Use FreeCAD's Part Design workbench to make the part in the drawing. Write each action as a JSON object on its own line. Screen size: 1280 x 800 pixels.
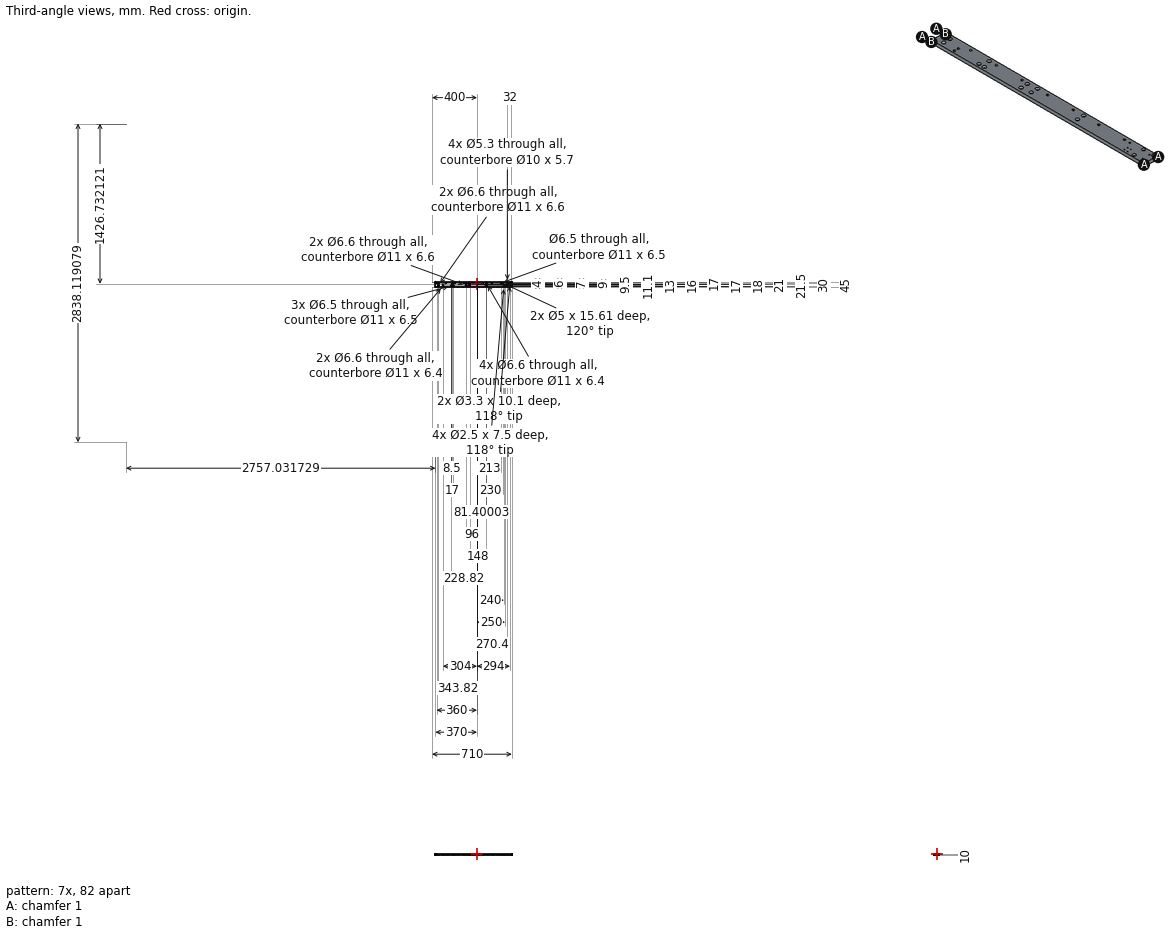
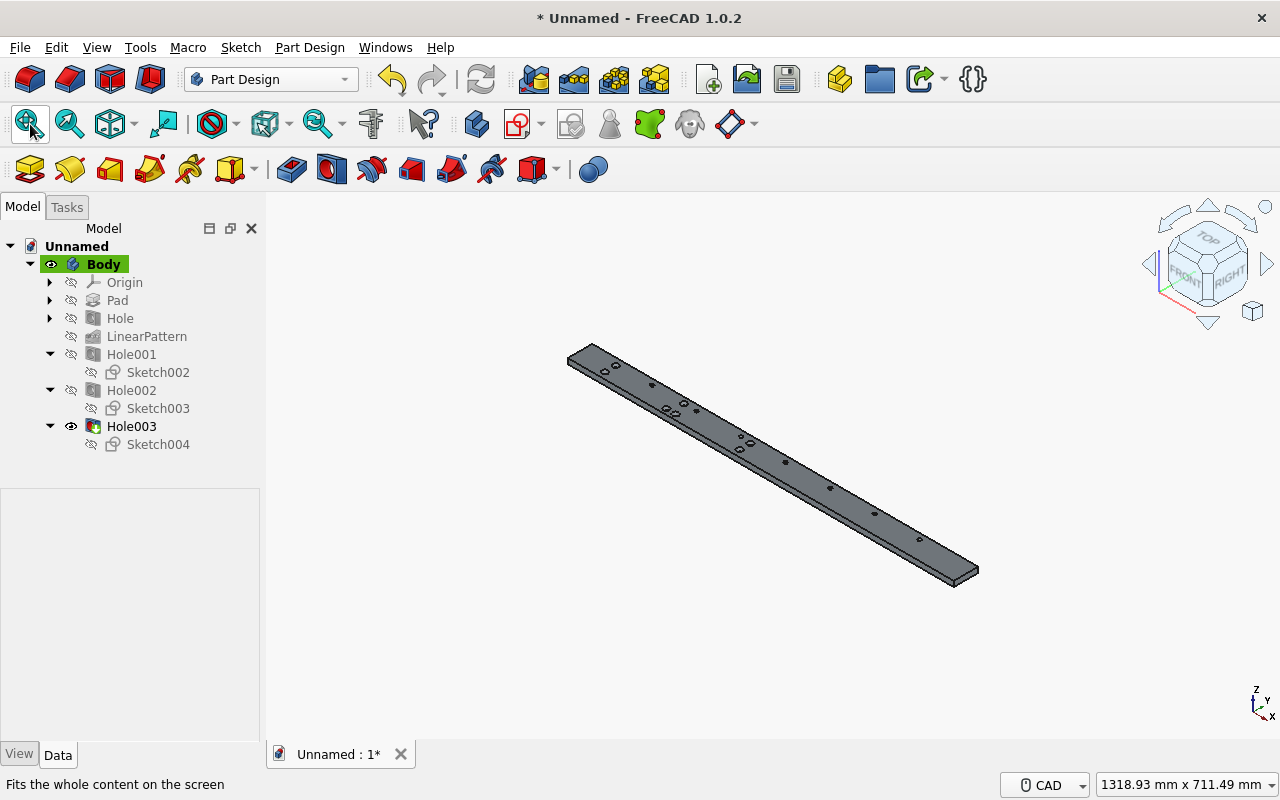
{"action": "key", "text": "5"}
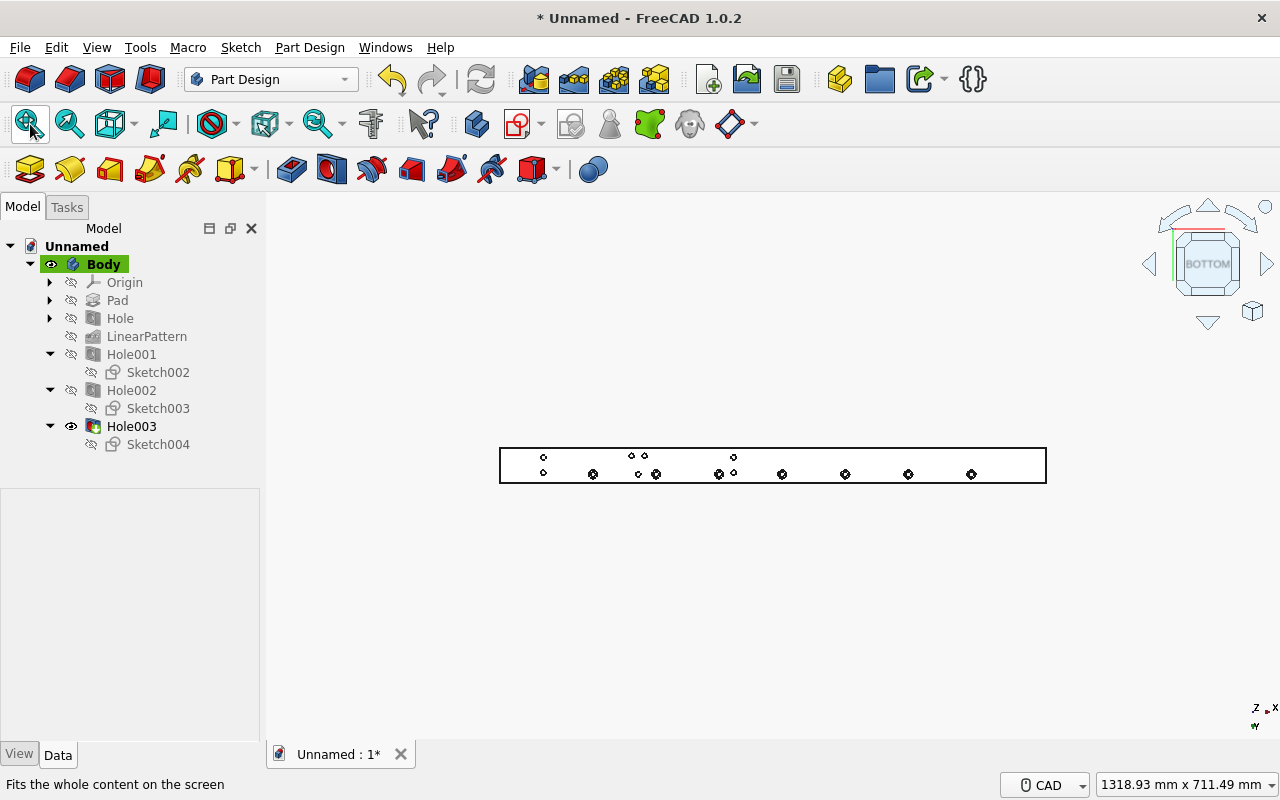
{"action": "left_click", "coordinate": [1007, 464]}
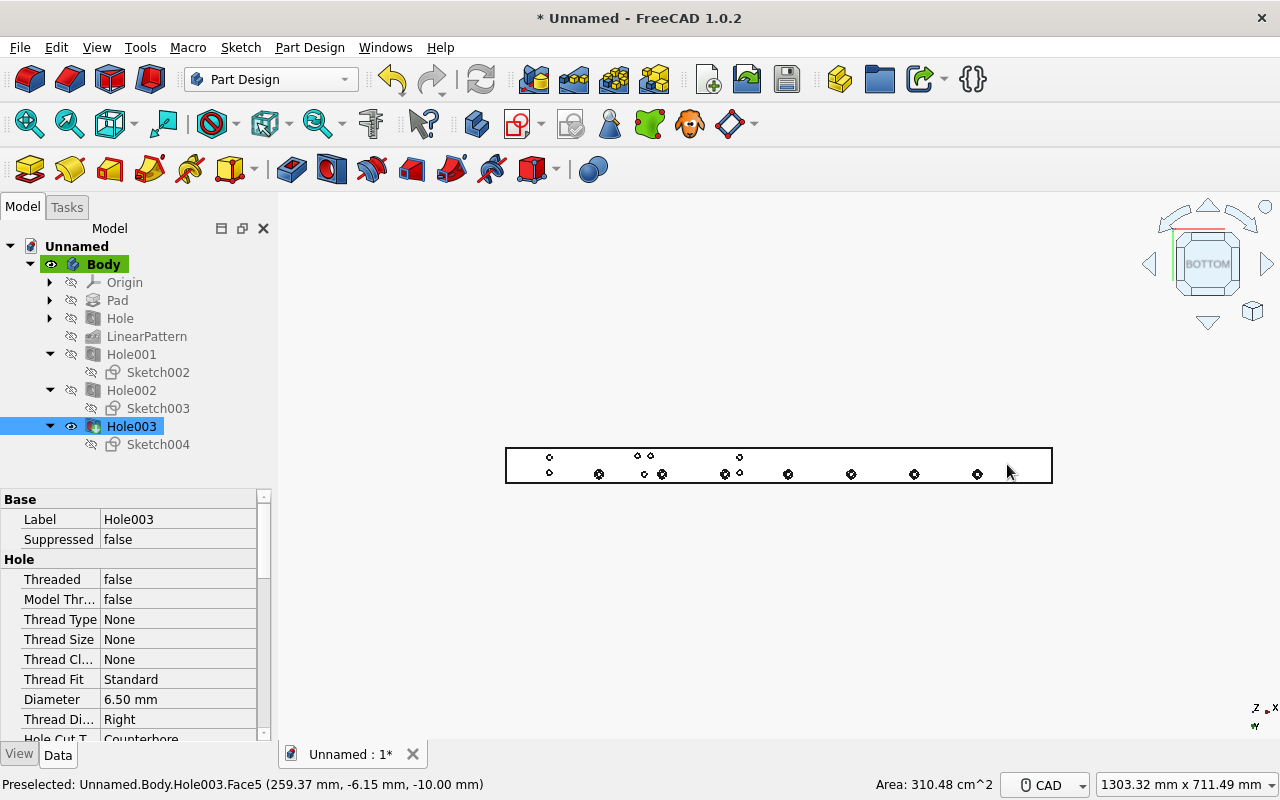
{"action": "left_click", "coordinate": [518, 124]}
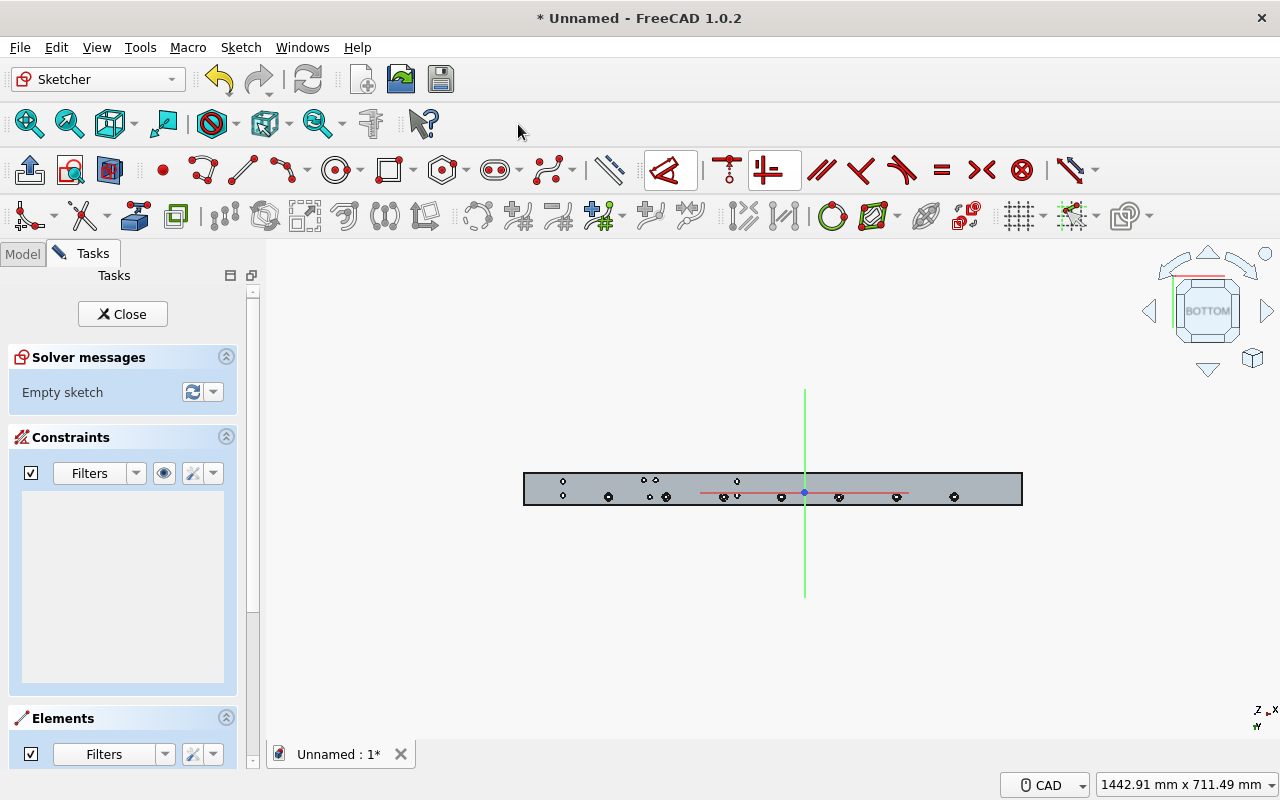
{"action": "scroll", "coordinate": [585, 482], "scroll_direction": "up", "scroll_amount": 15}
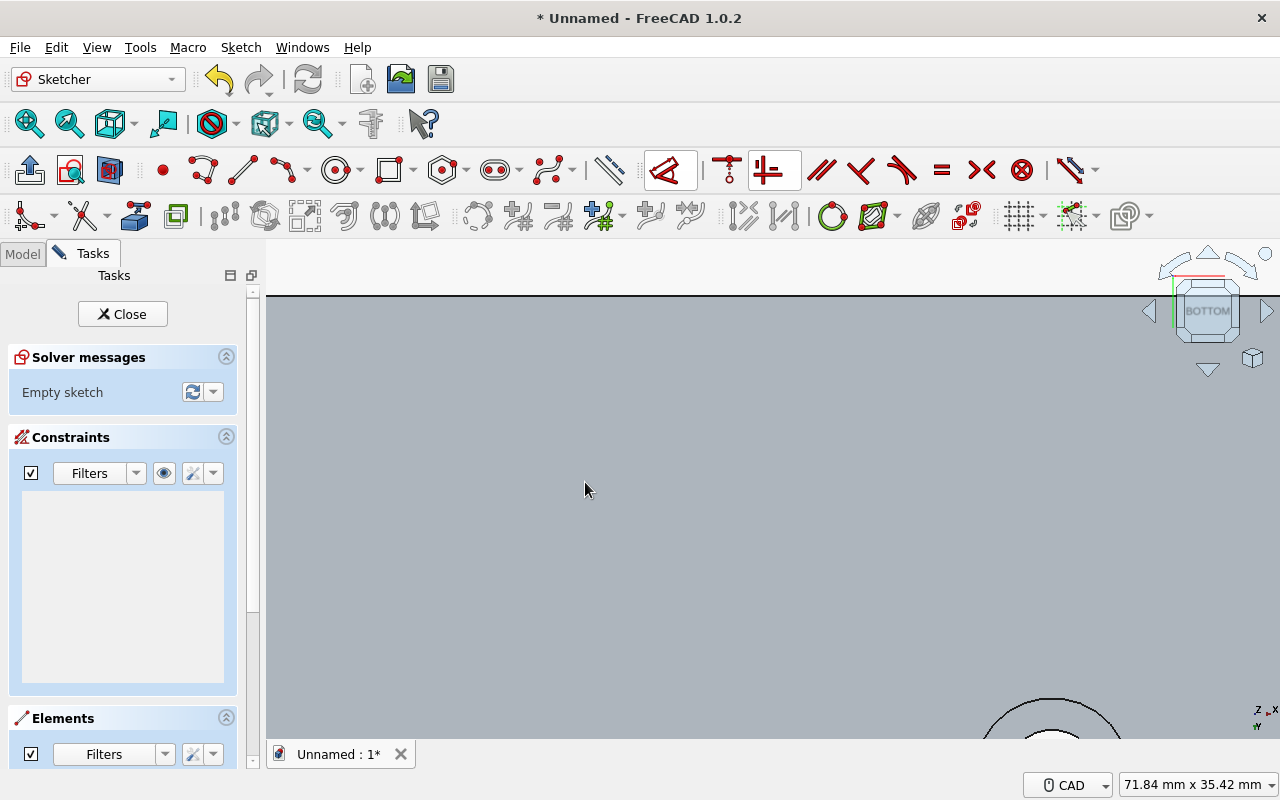
{"action": "left_click", "coordinate": [336, 170]}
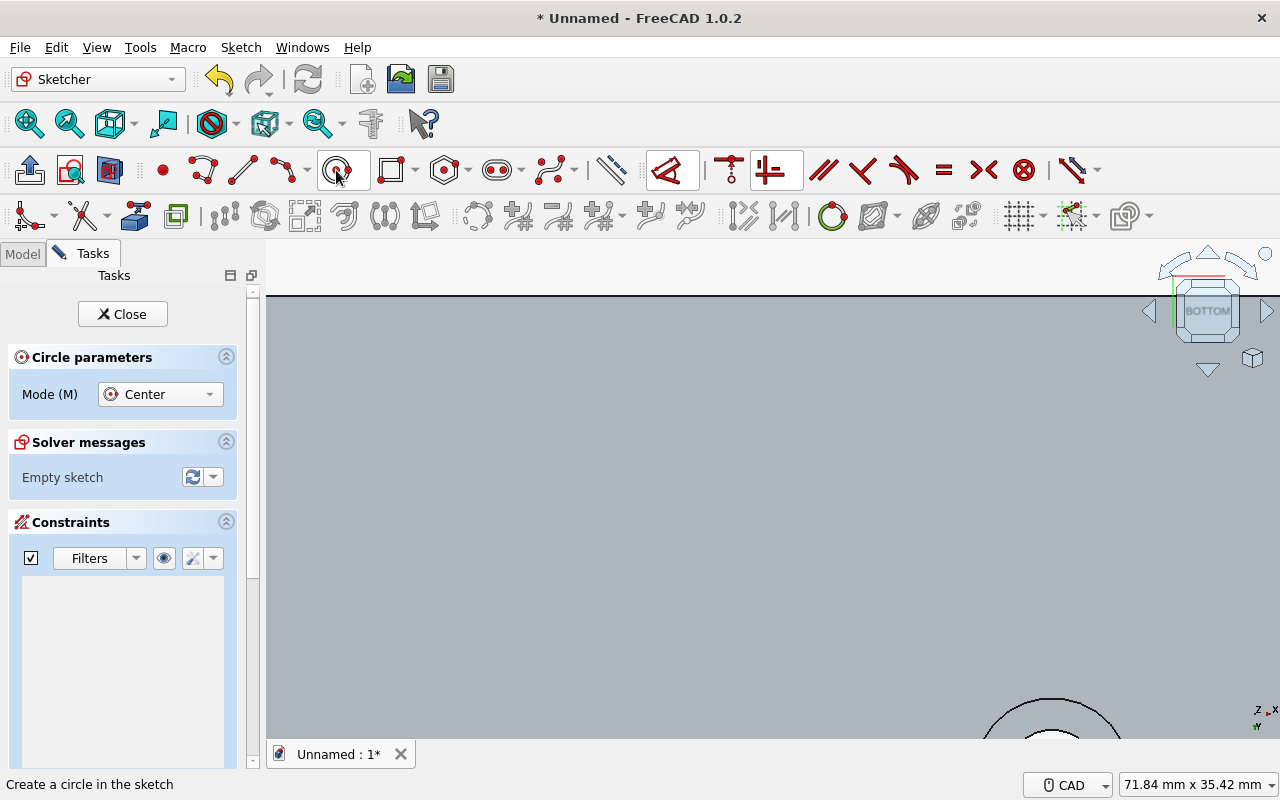
{"action": "left_click", "coordinate": [699, 395]}
{"action": "left_click", "coordinate": [732, 362]}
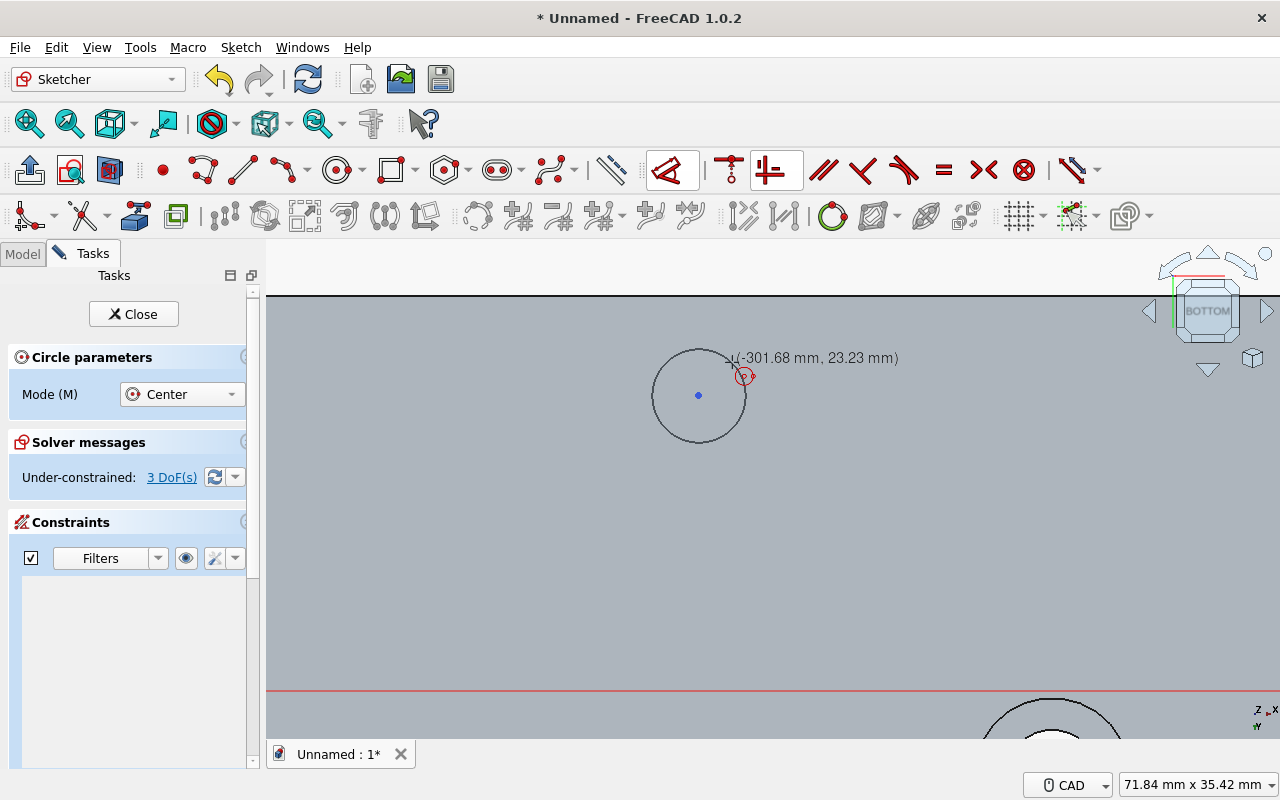
{"action": "left_click", "coordinate": [699, 564]}
{"action": "left_click", "coordinate": [732, 531]}
{"action": "key", "text": "Escape"}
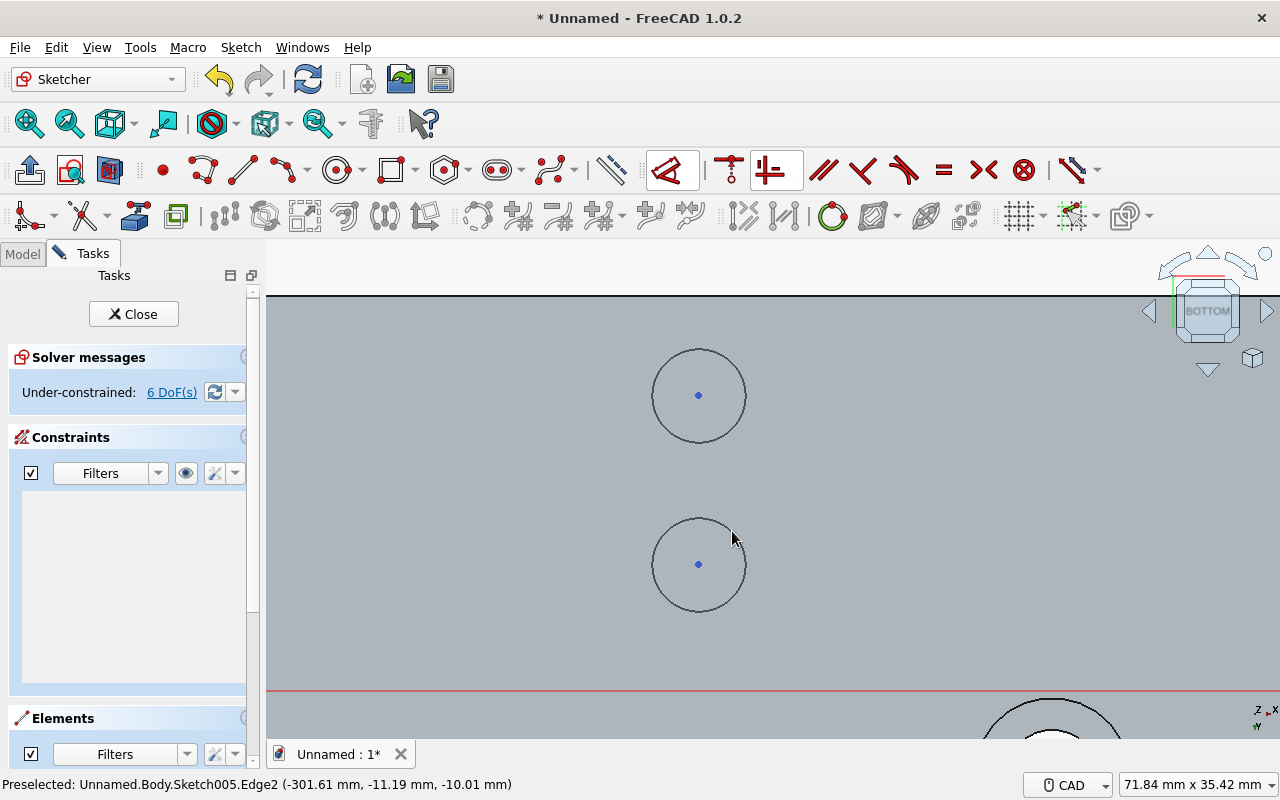
{"action": "left_click", "coordinate": [732, 363]}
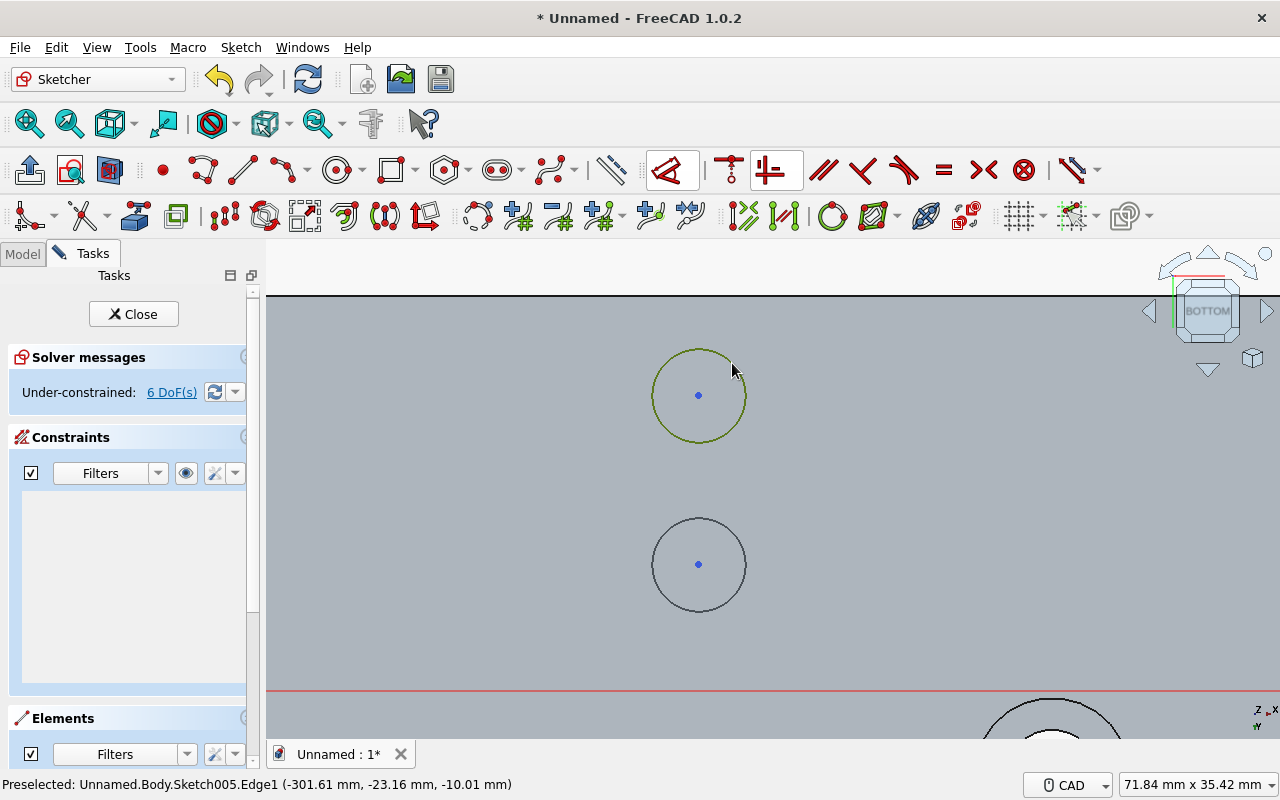
{"action": "left_click", "coordinate": [732, 532]}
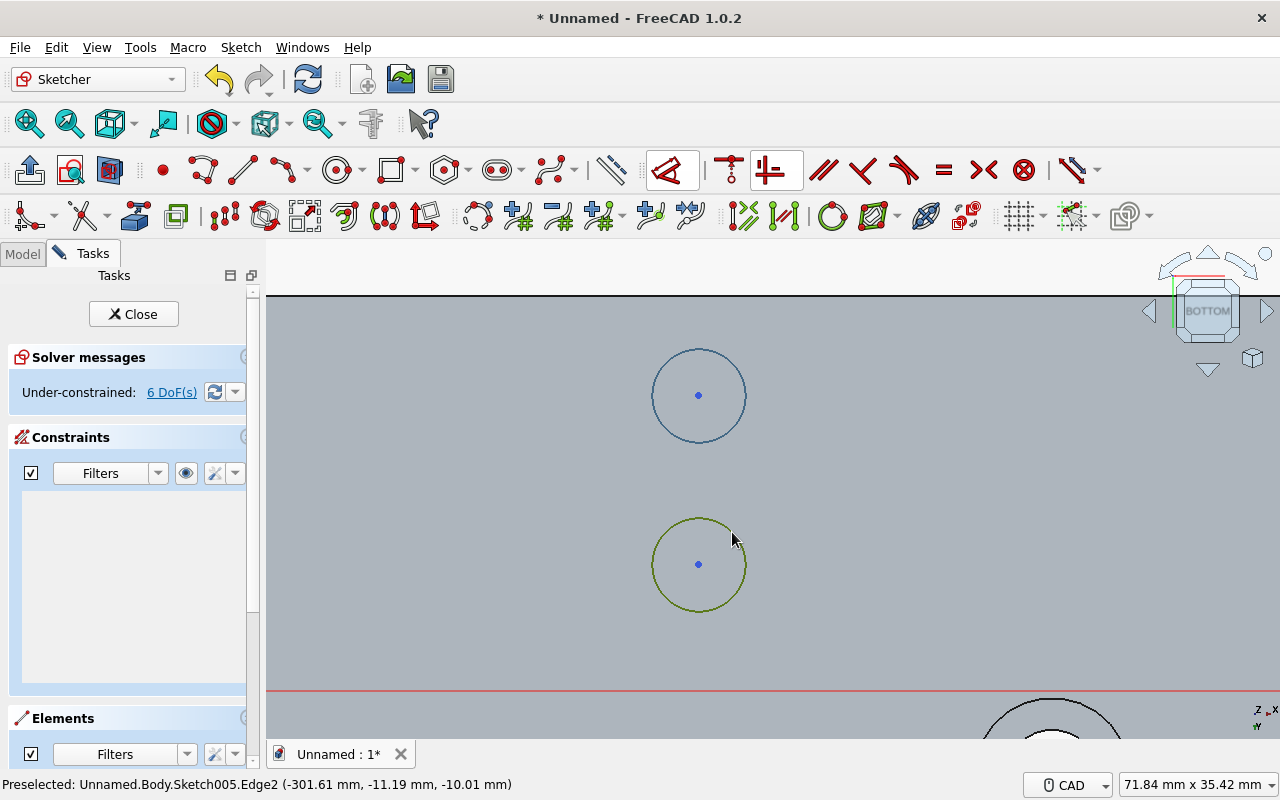
{"action": "left_click", "coordinate": [944, 170]}